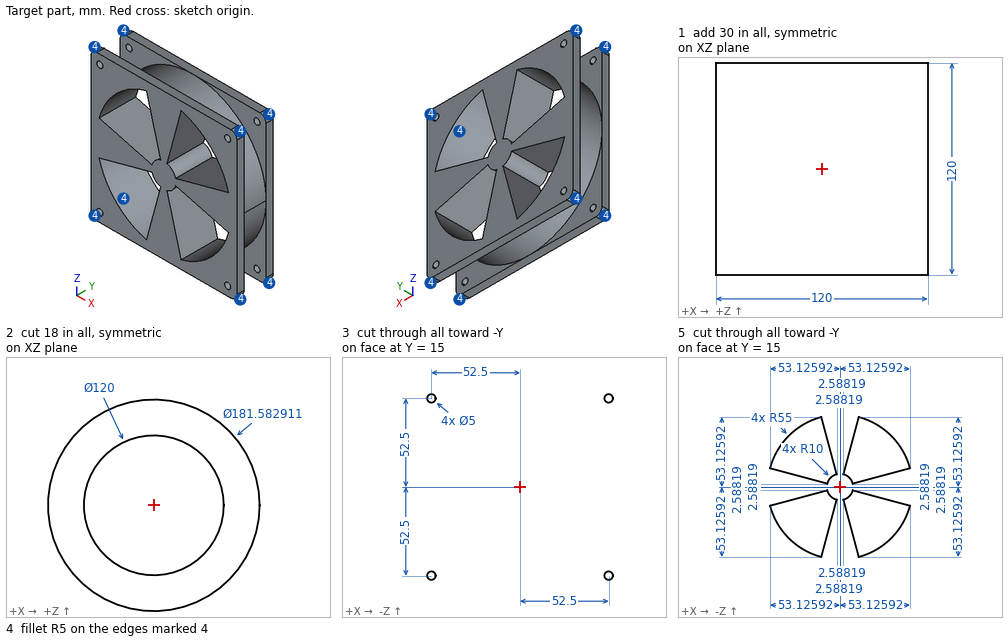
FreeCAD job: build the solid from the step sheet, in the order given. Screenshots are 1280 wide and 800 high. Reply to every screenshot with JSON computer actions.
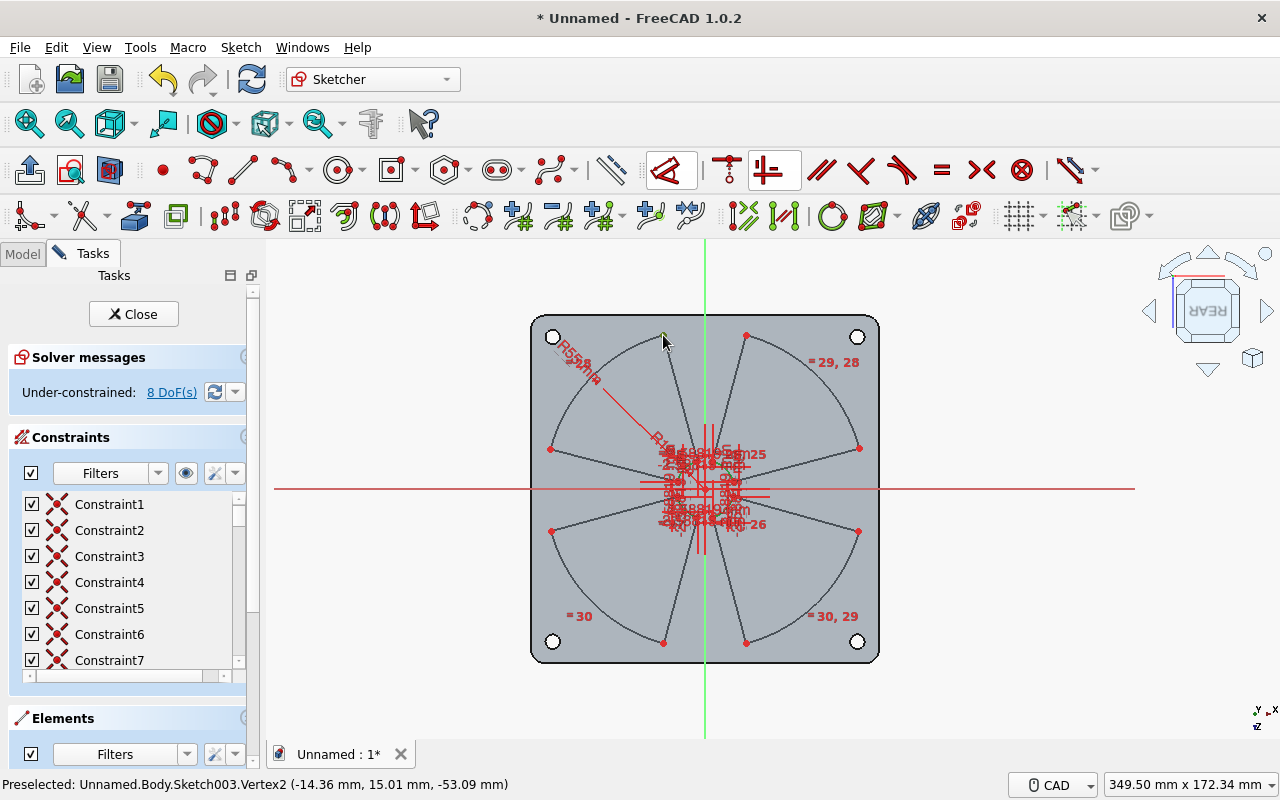
{"action": "left_click", "coordinate": [692, 170]}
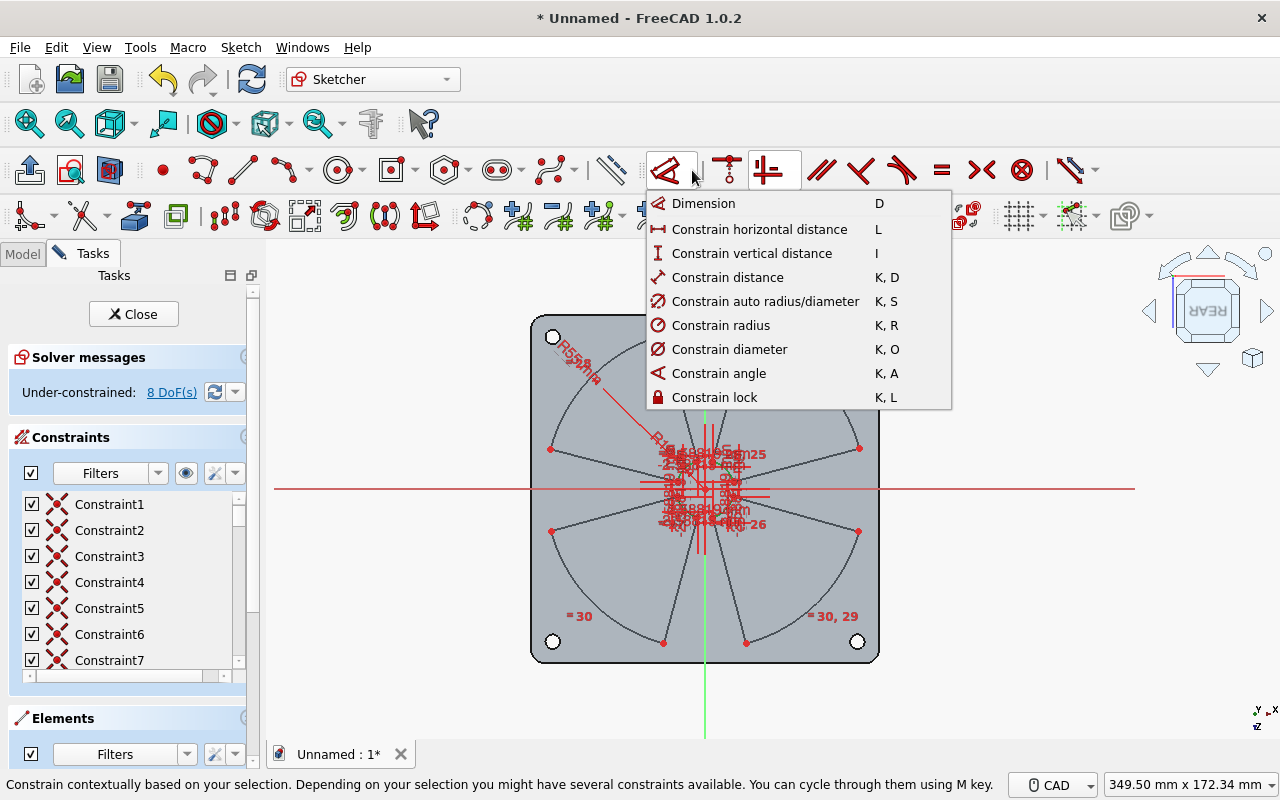
{"action": "left_click", "coordinate": [799, 253]}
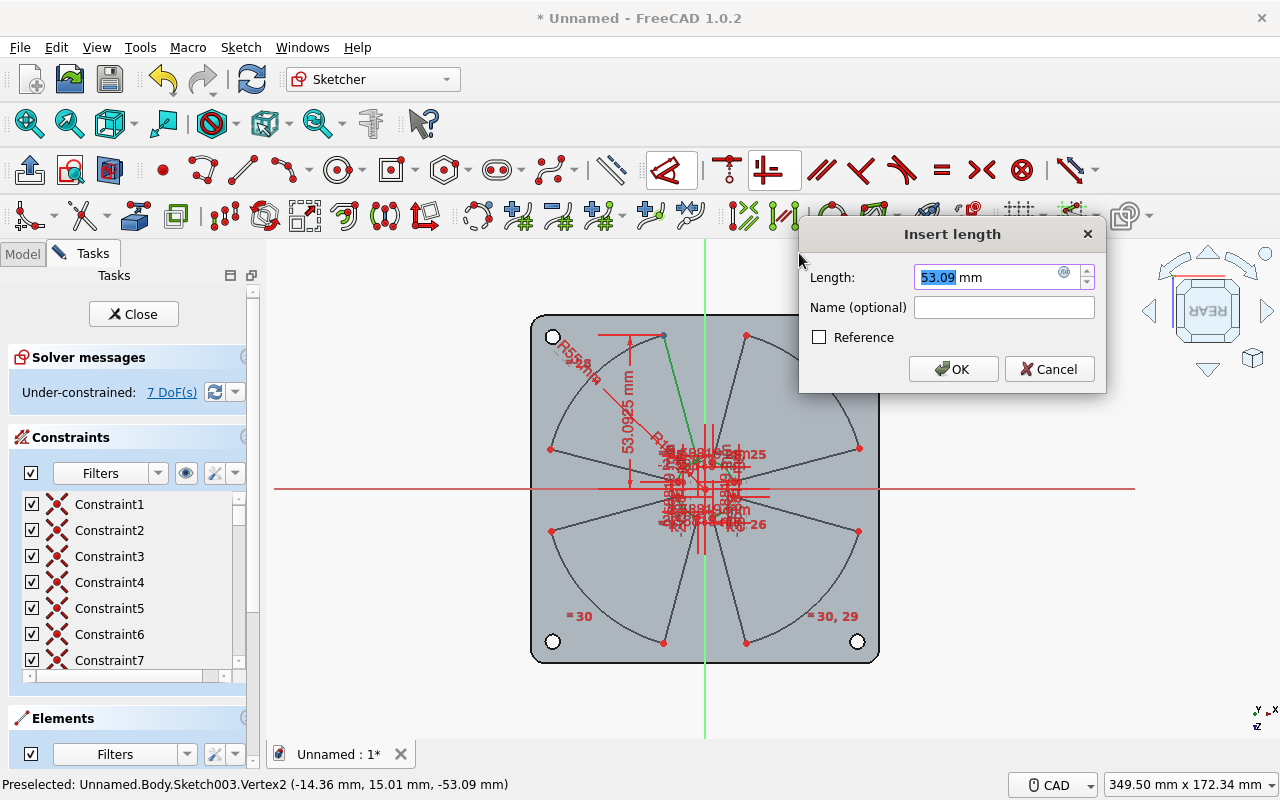
{"action": "type", "text": "53.12592"}
{"action": "key", "text": "Return"}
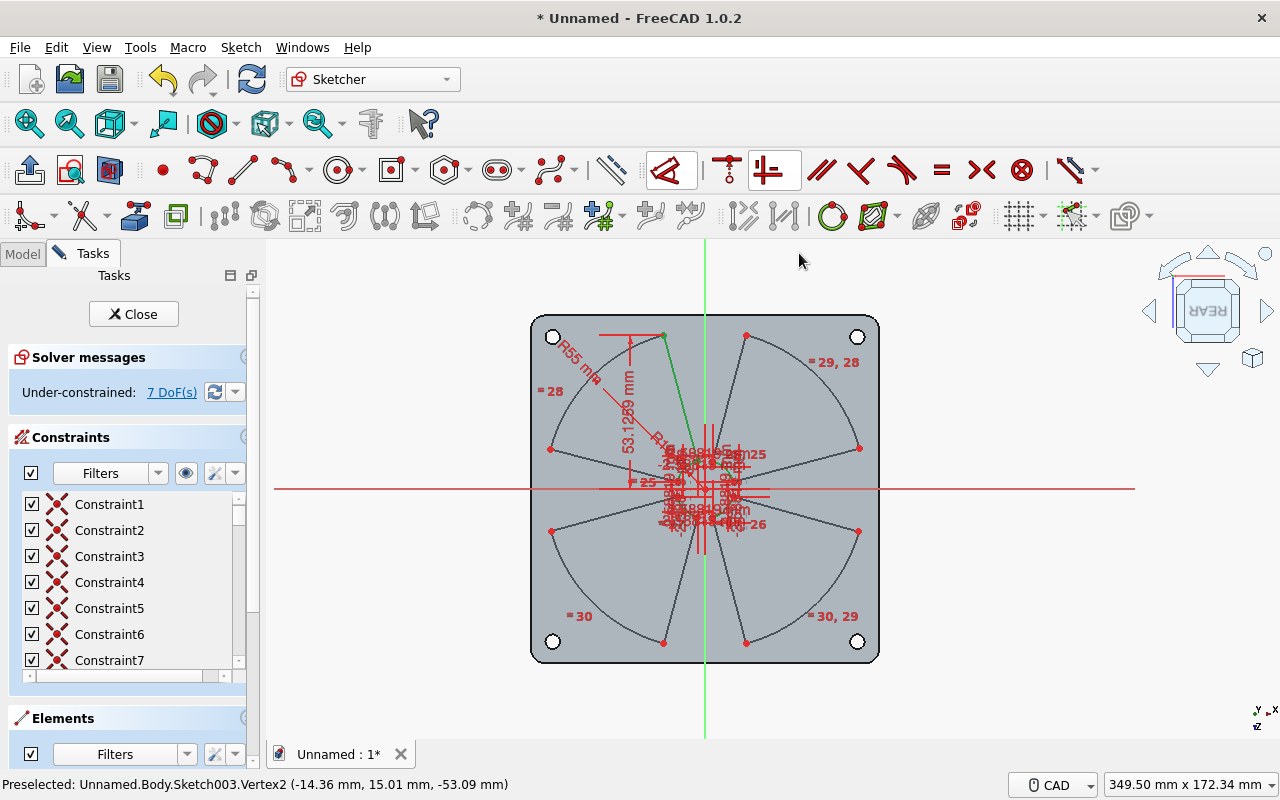
{"action": "left_click", "coordinate": [551, 449]}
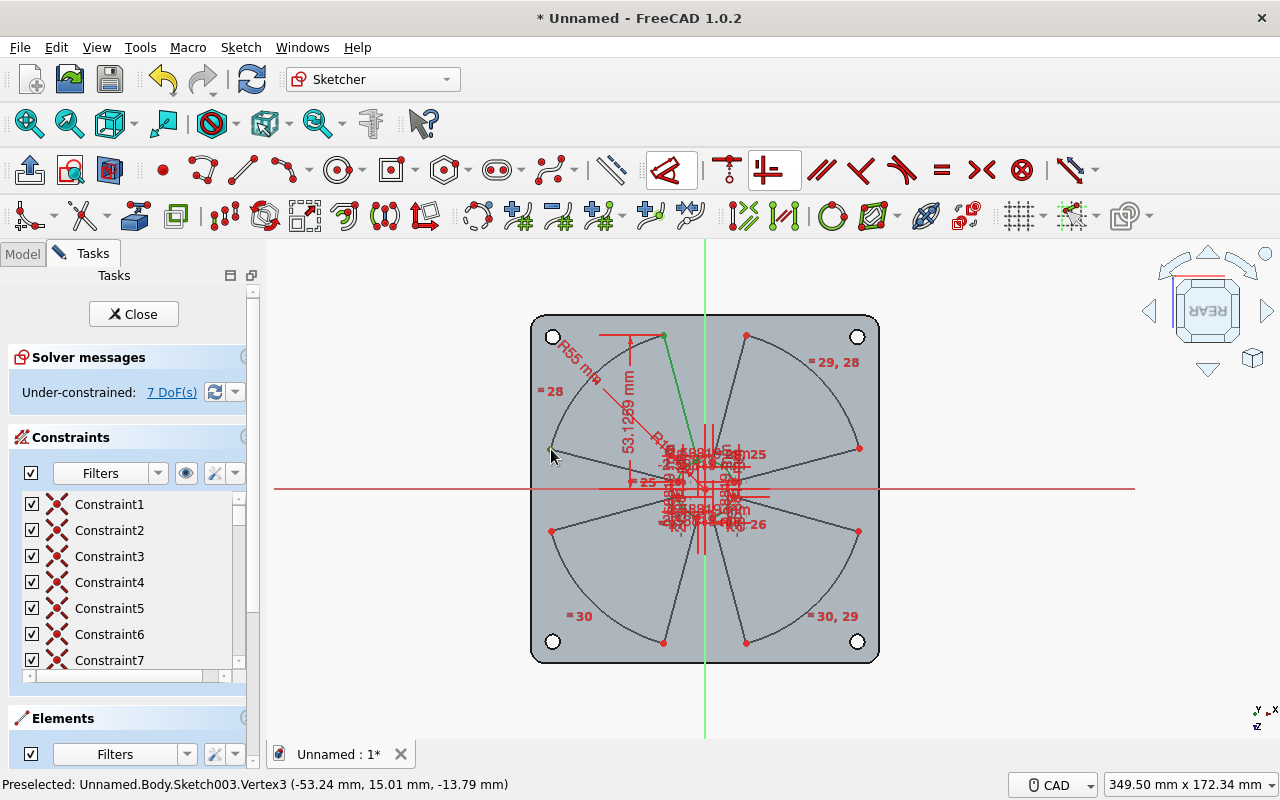
{"action": "key", "text": "l"}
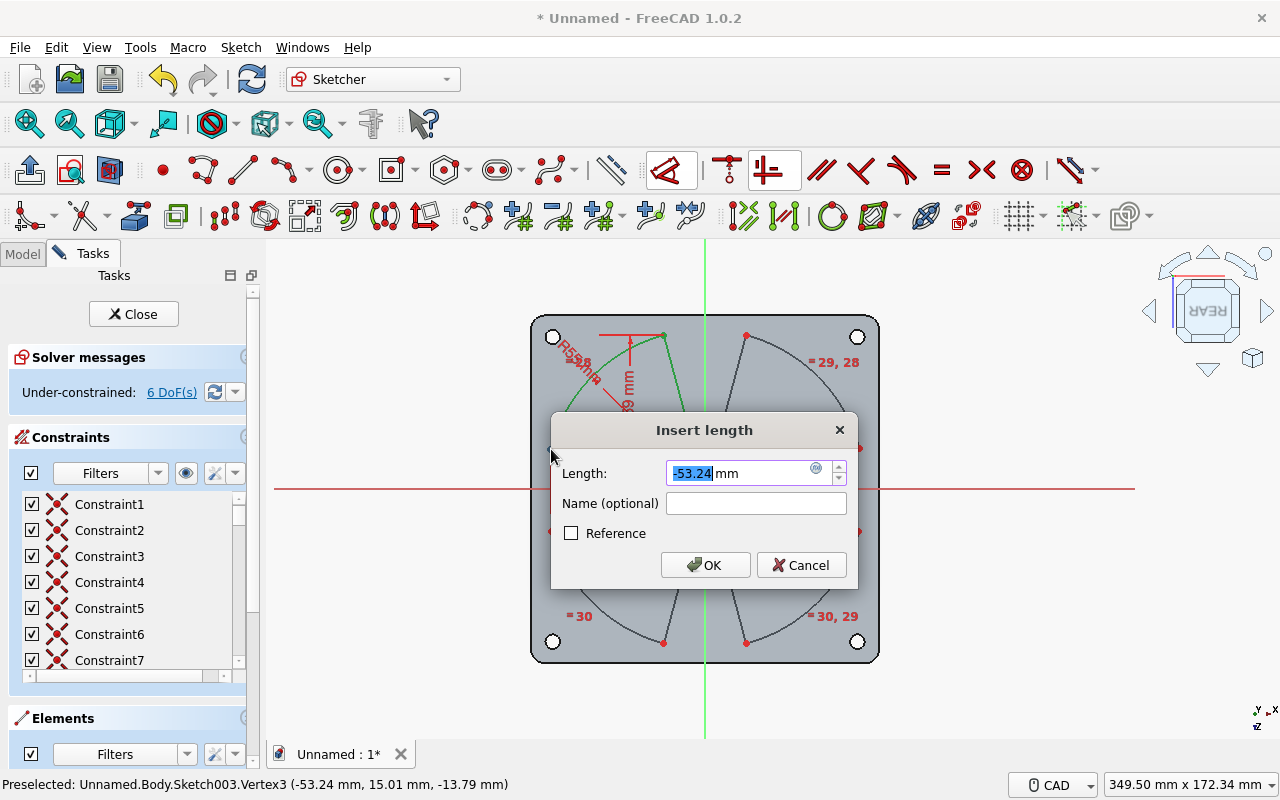
{"action": "type", "text": "-53.12592"}
{"action": "key", "text": "Return"}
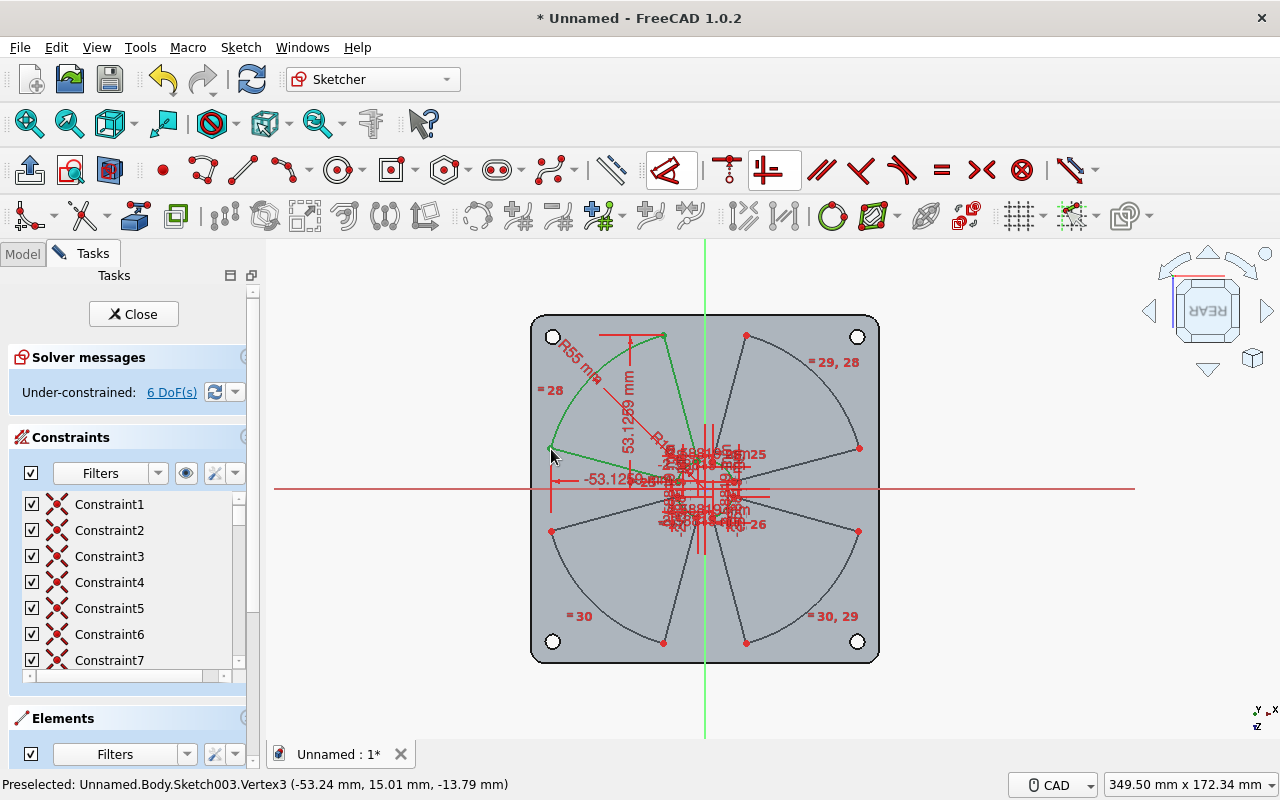
{"action": "left_click", "coordinate": [746, 335]}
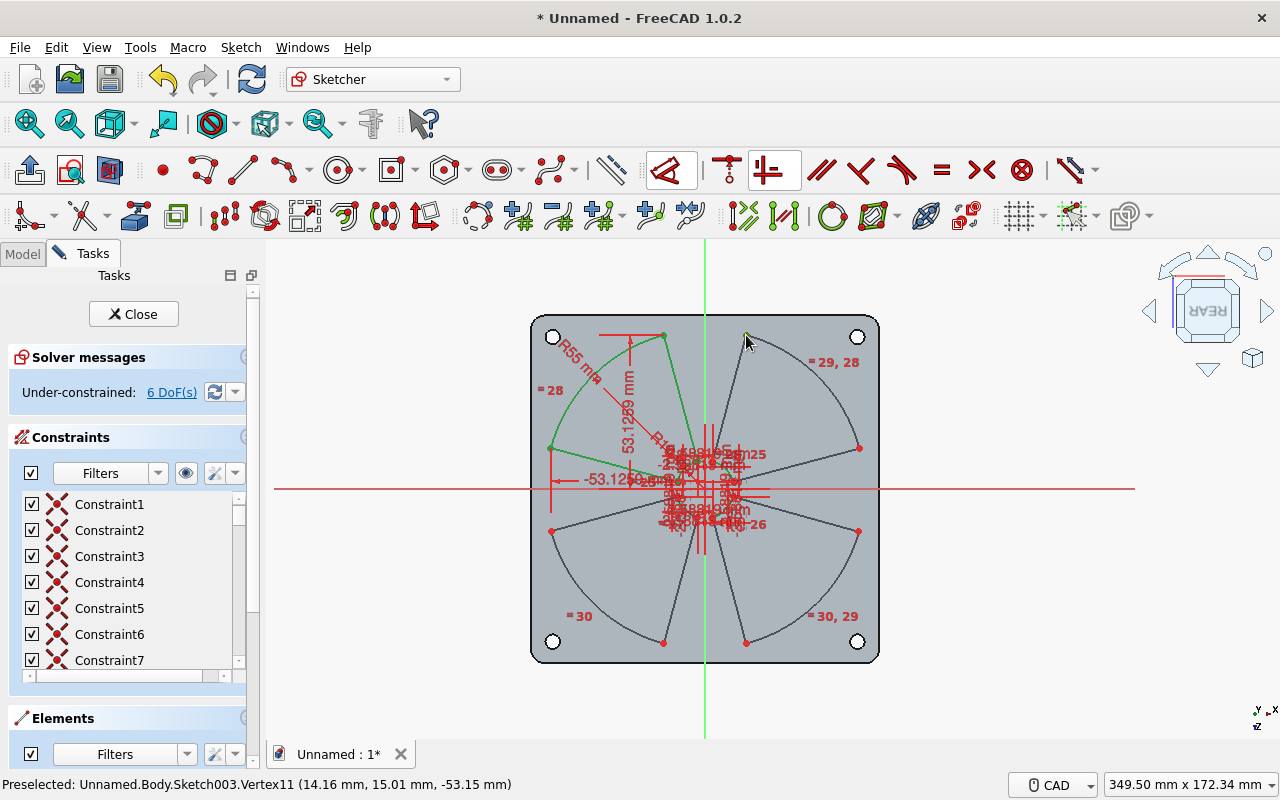
{"action": "left_click", "coordinate": [692, 170]}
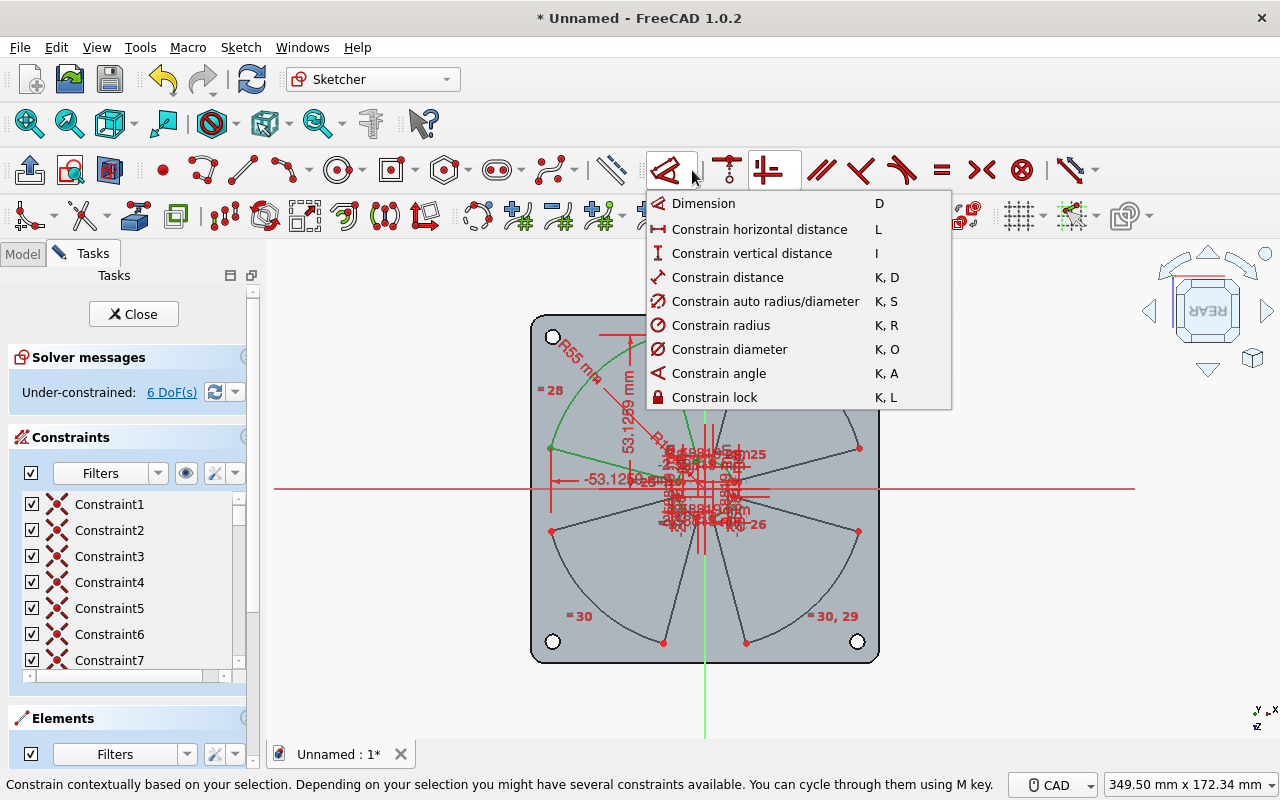
{"action": "left_click", "coordinate": [799, 253]}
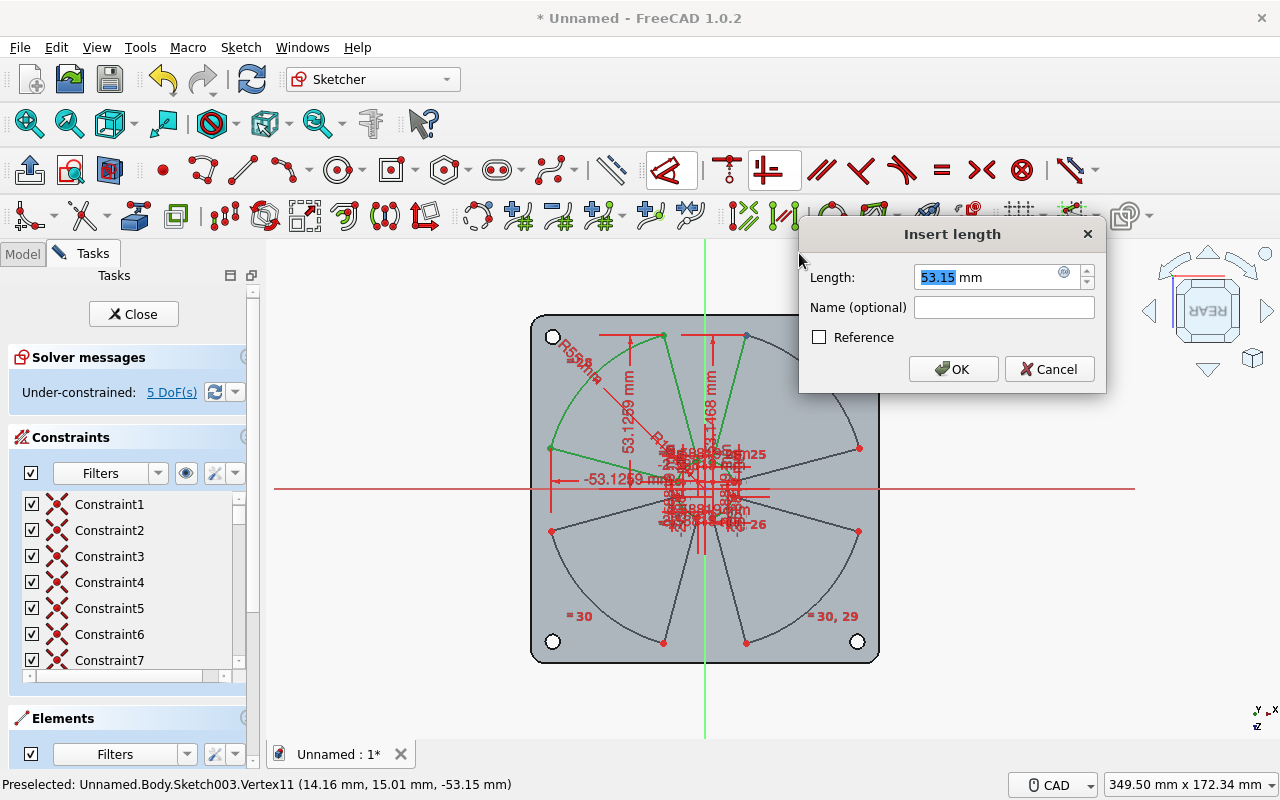
{"action": "type", "text": "53.12592"}
{"action": "key", "text": "Return"}